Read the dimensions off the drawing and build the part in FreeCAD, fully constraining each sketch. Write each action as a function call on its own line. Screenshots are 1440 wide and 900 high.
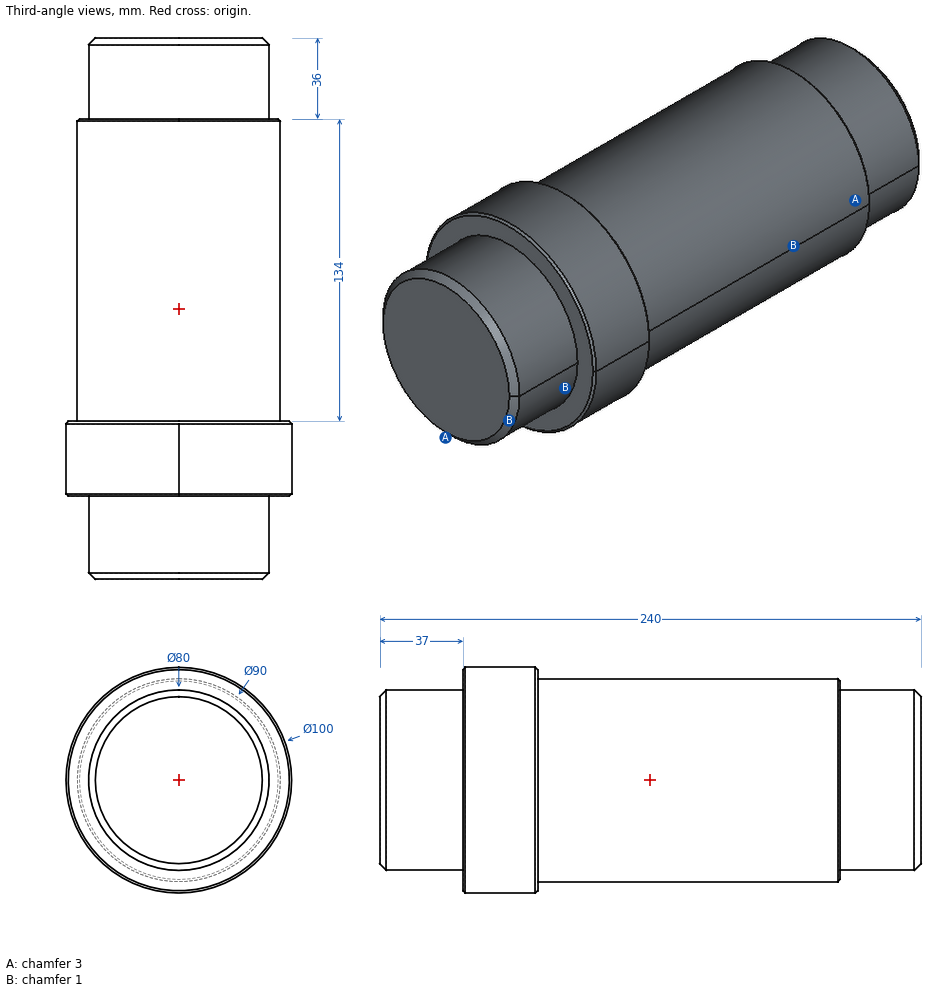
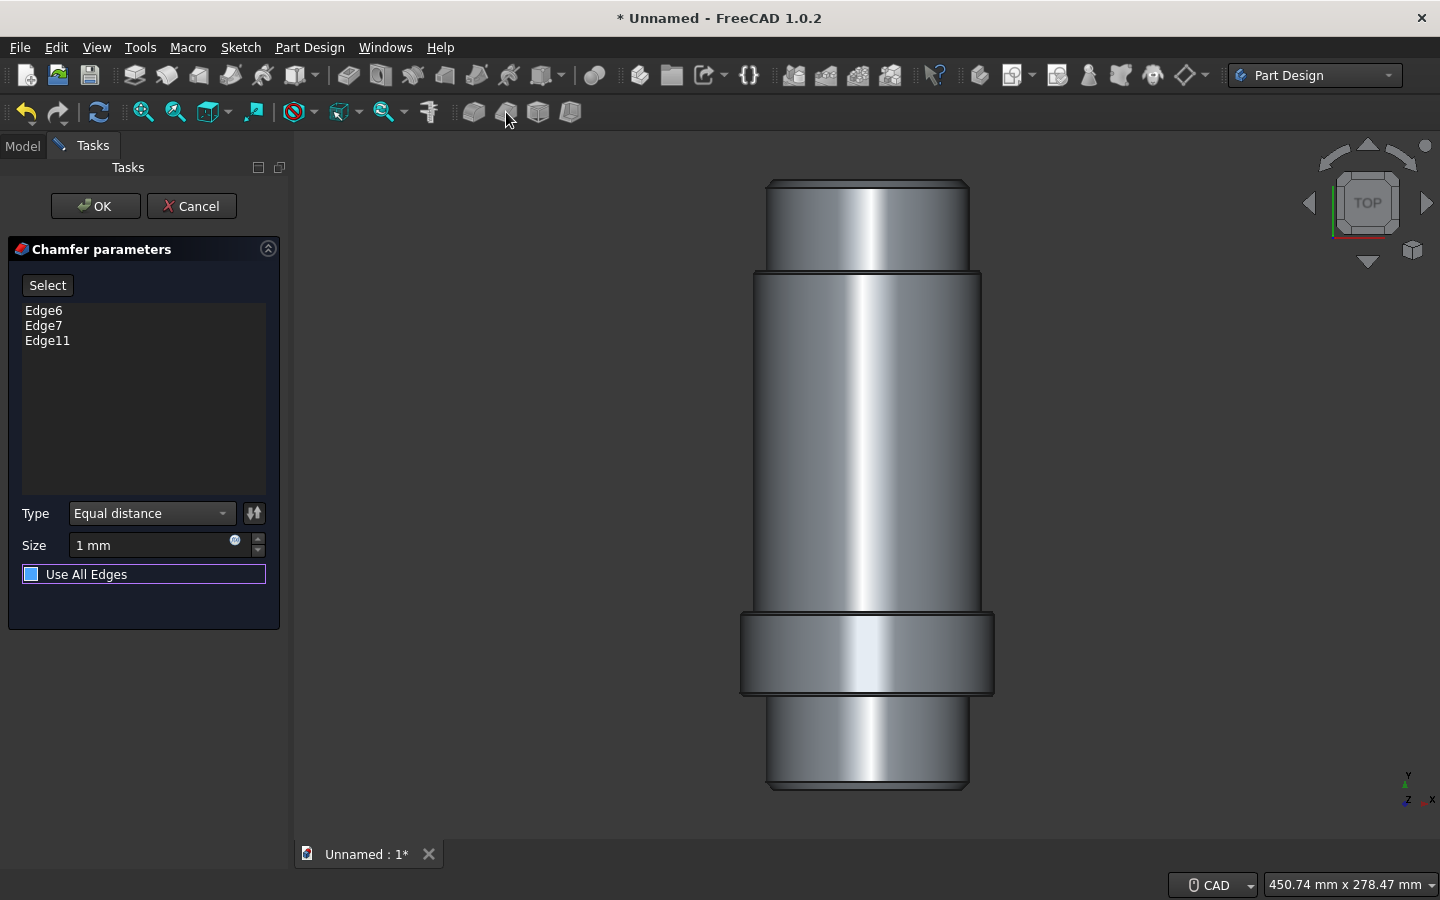
click(96, 206)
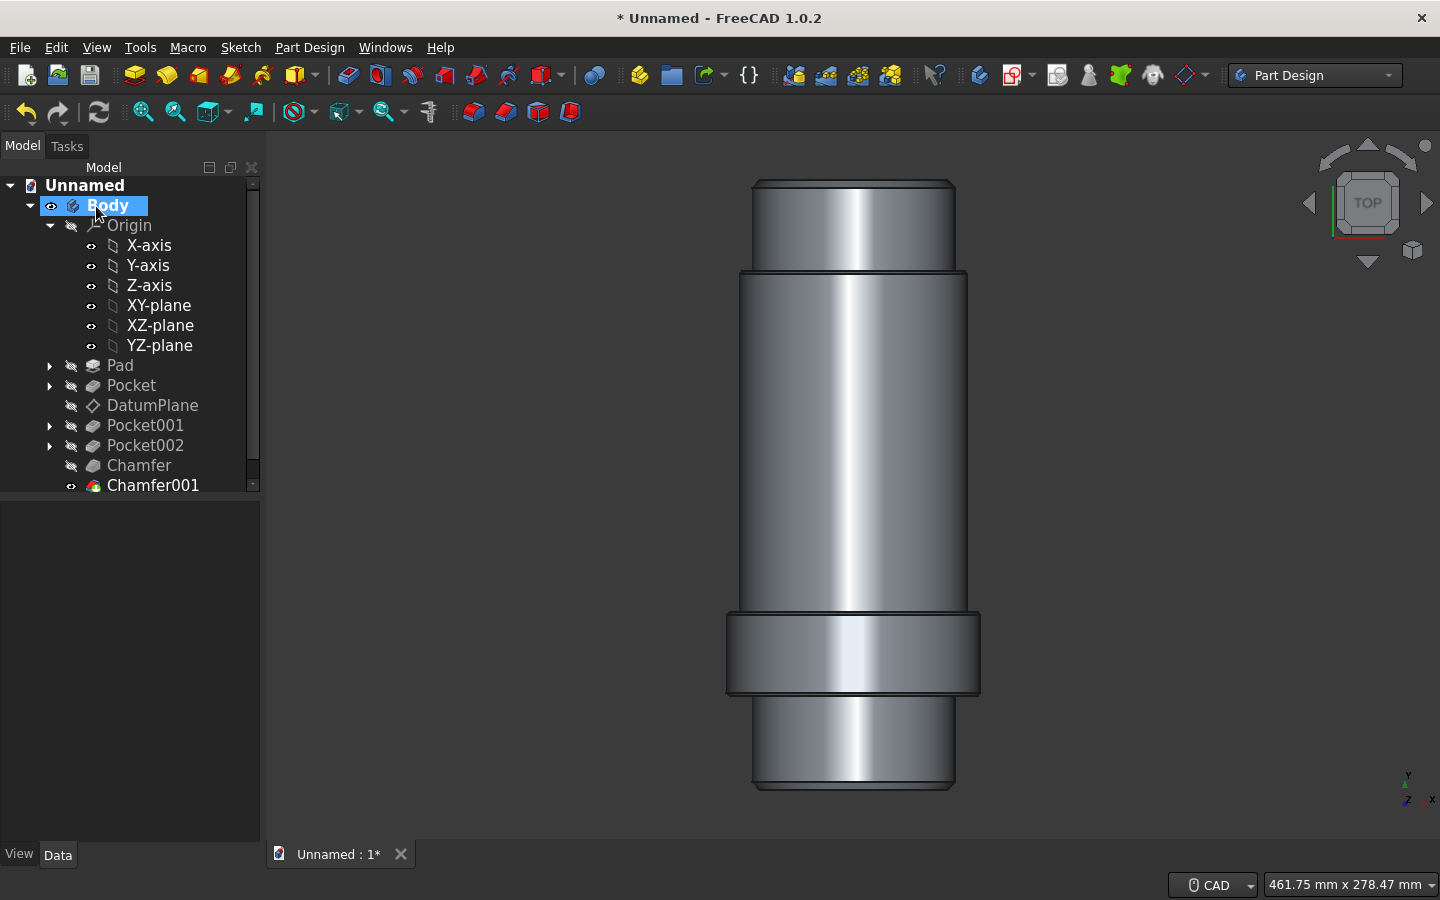
key(0)